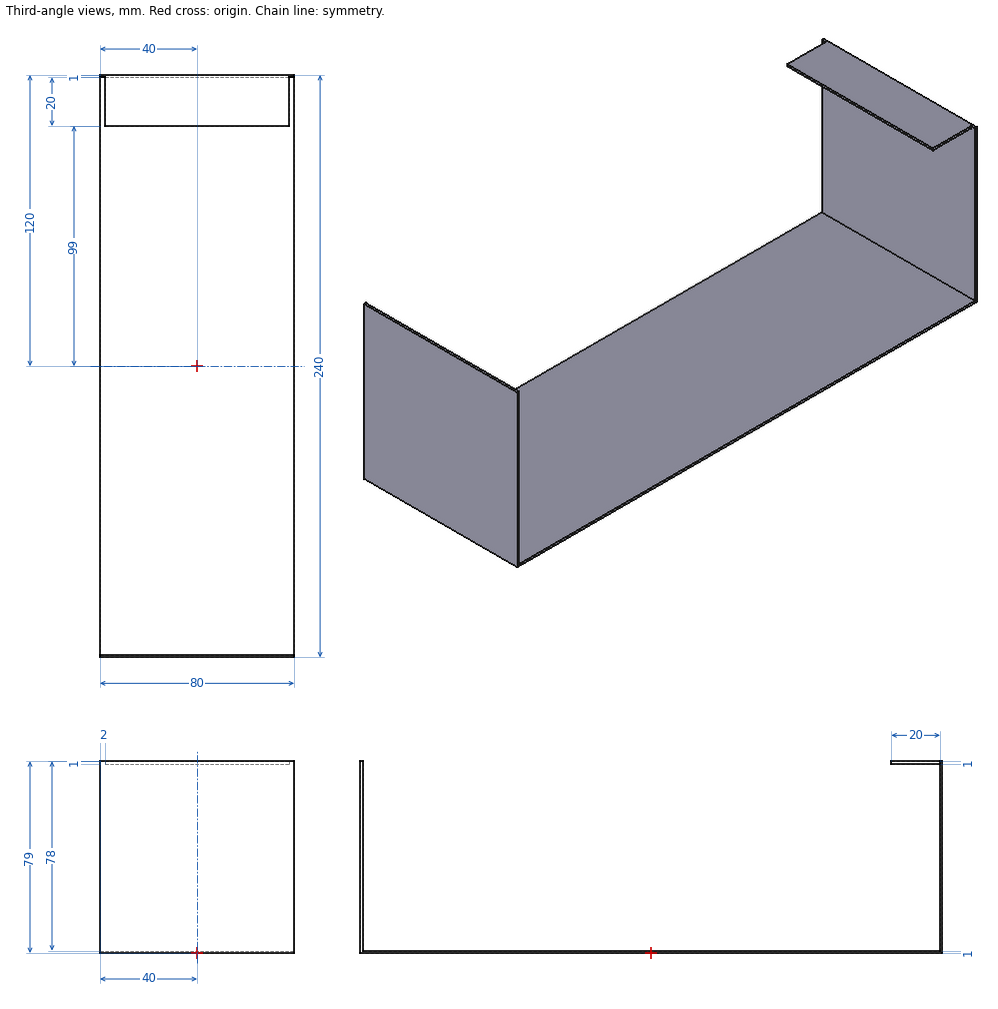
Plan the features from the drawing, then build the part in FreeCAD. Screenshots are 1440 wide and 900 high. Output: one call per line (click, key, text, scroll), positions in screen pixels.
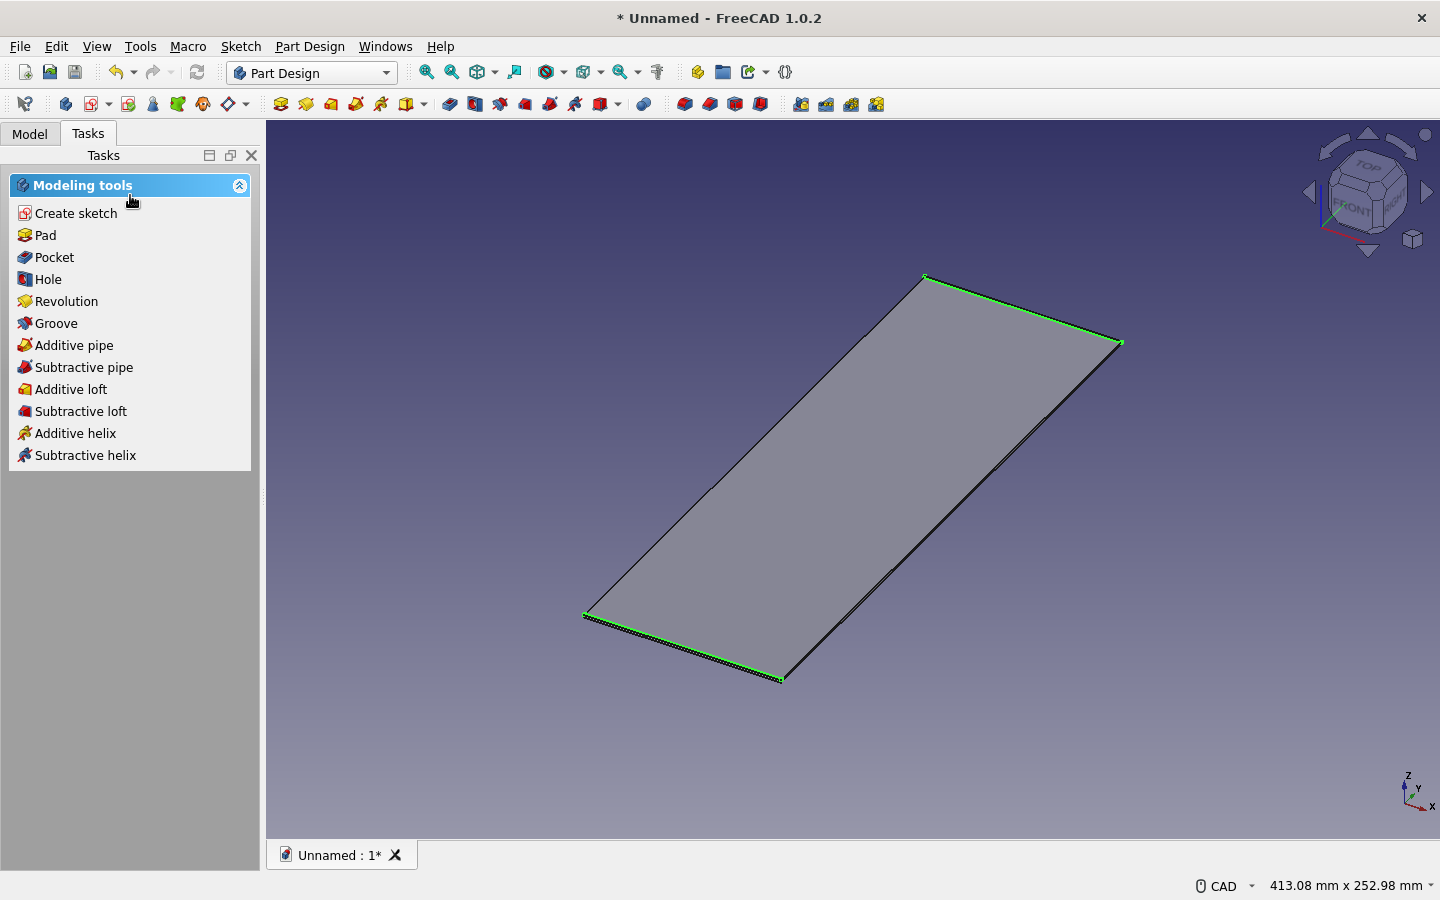
click(281, 104)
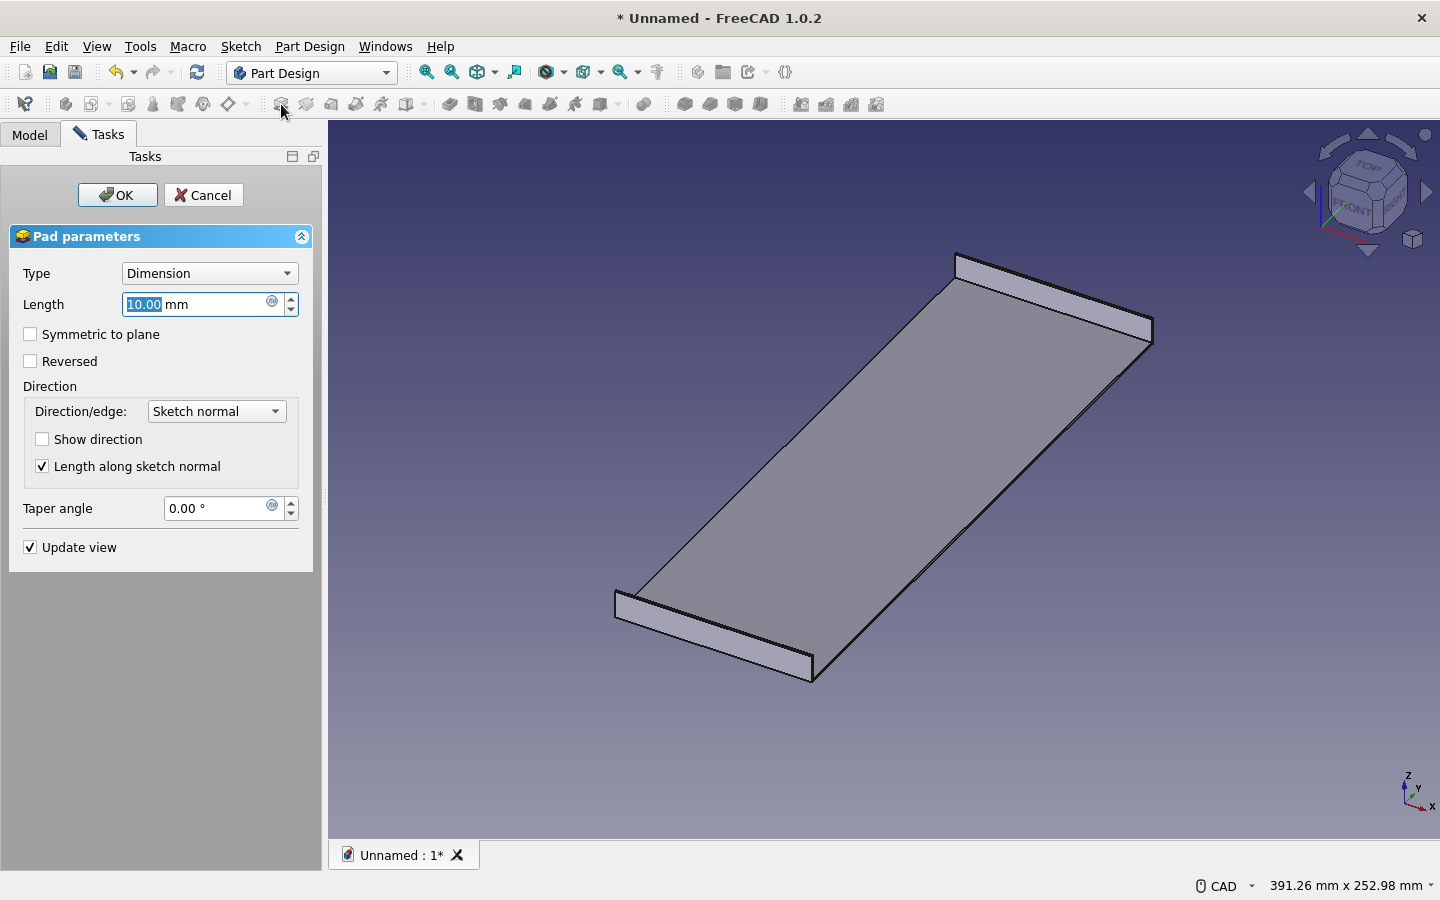
text(78)
key(Tab)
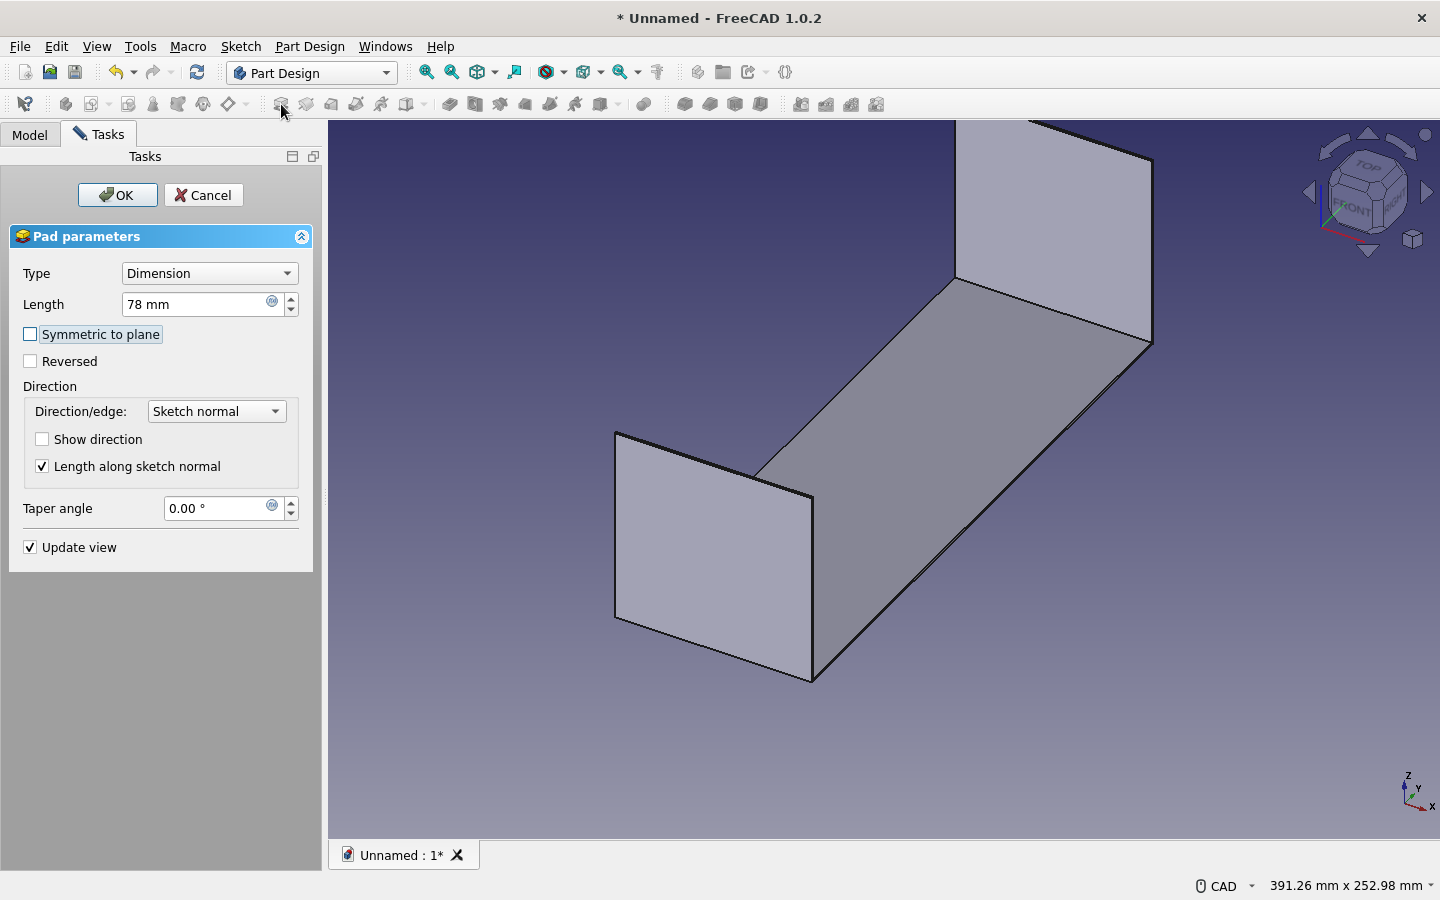
click(118, 195)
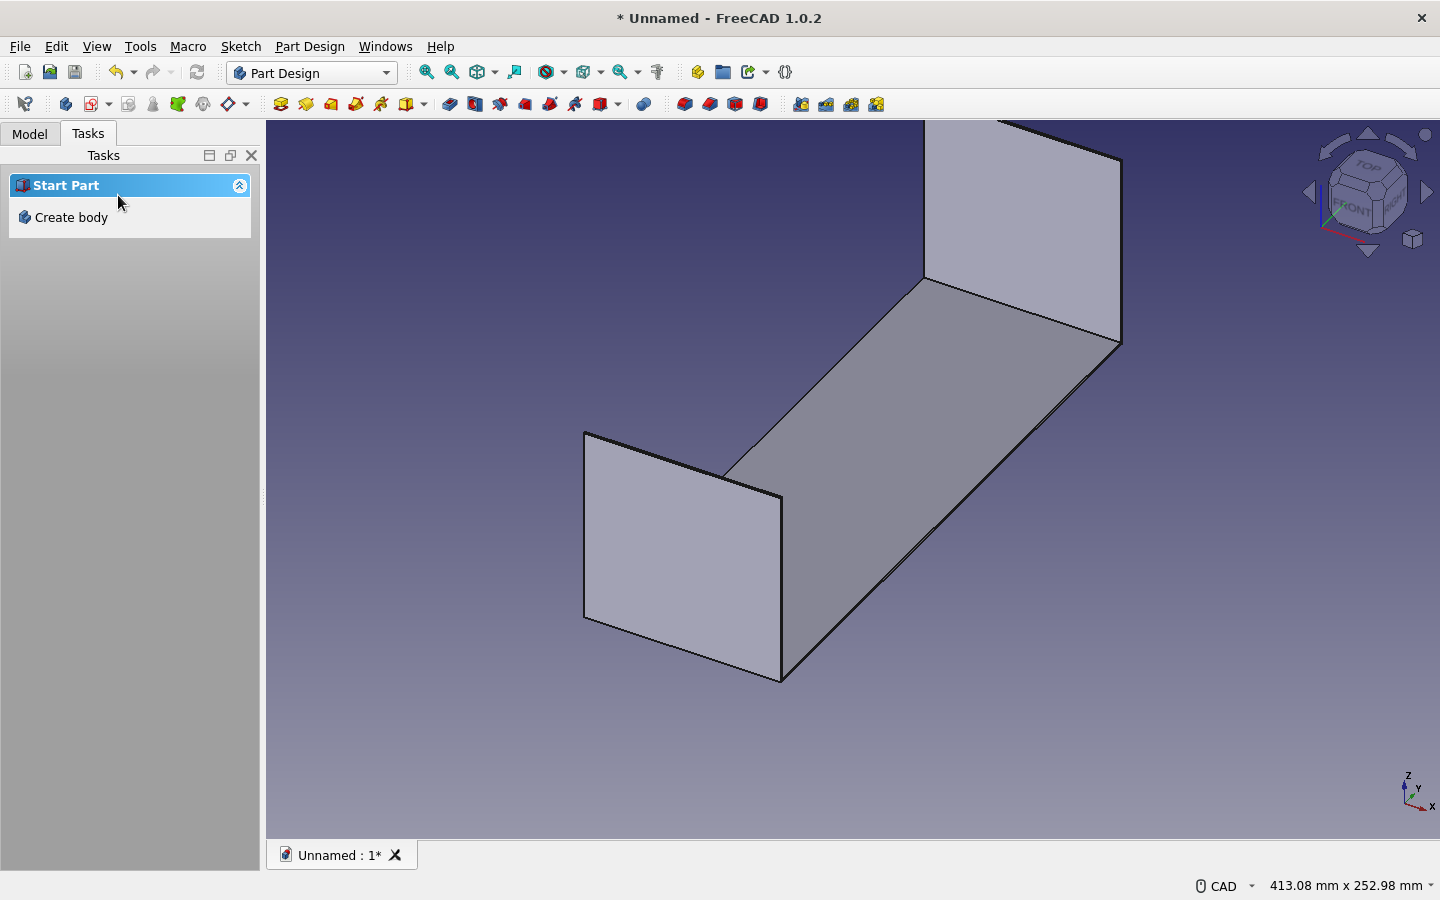
key(v)
key(f)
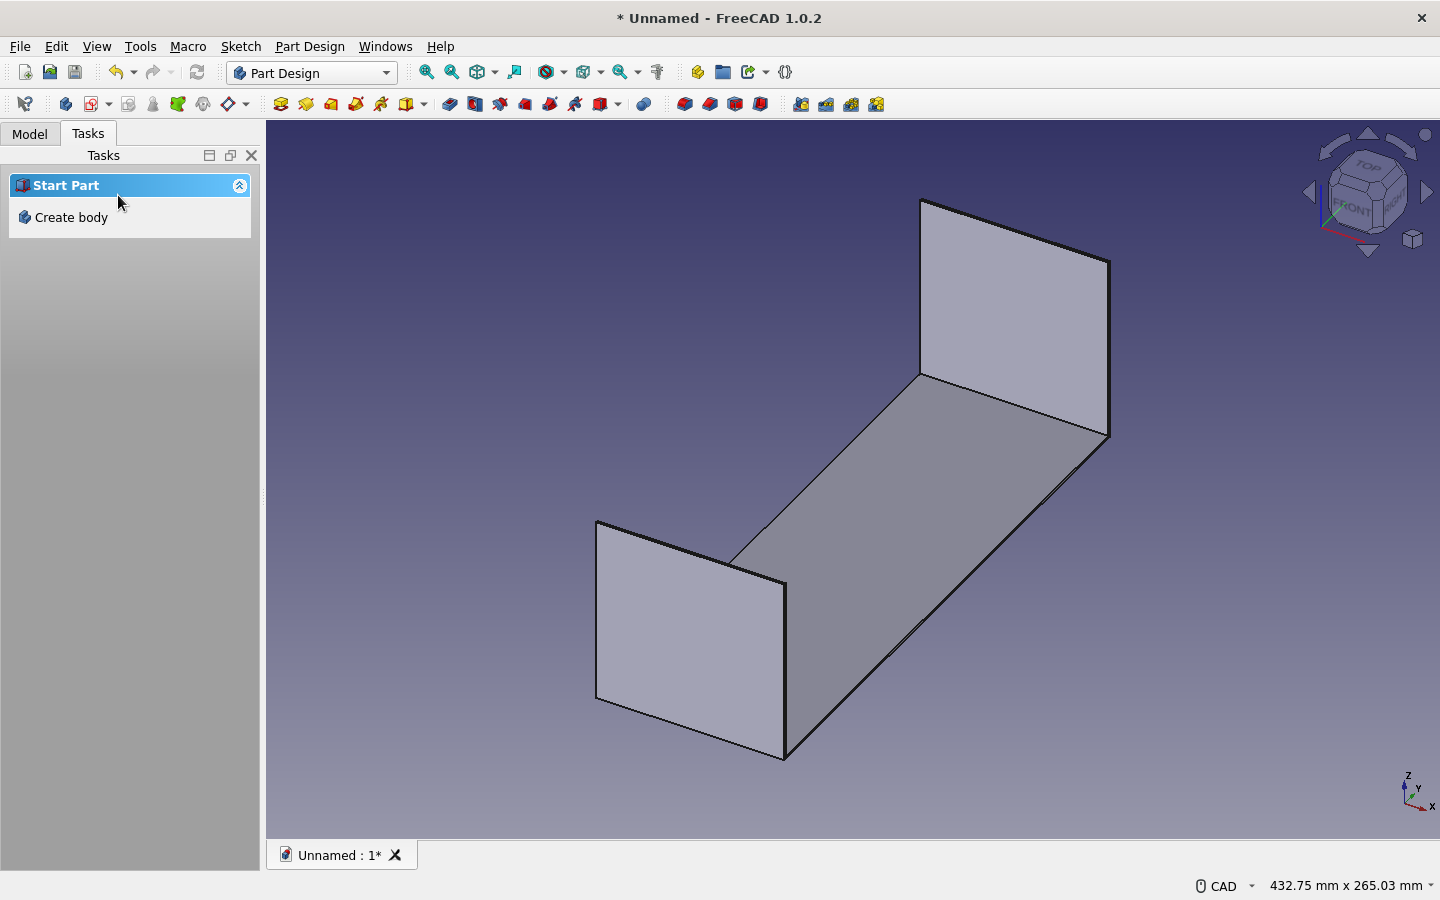
scroll(771, 578, up, 11)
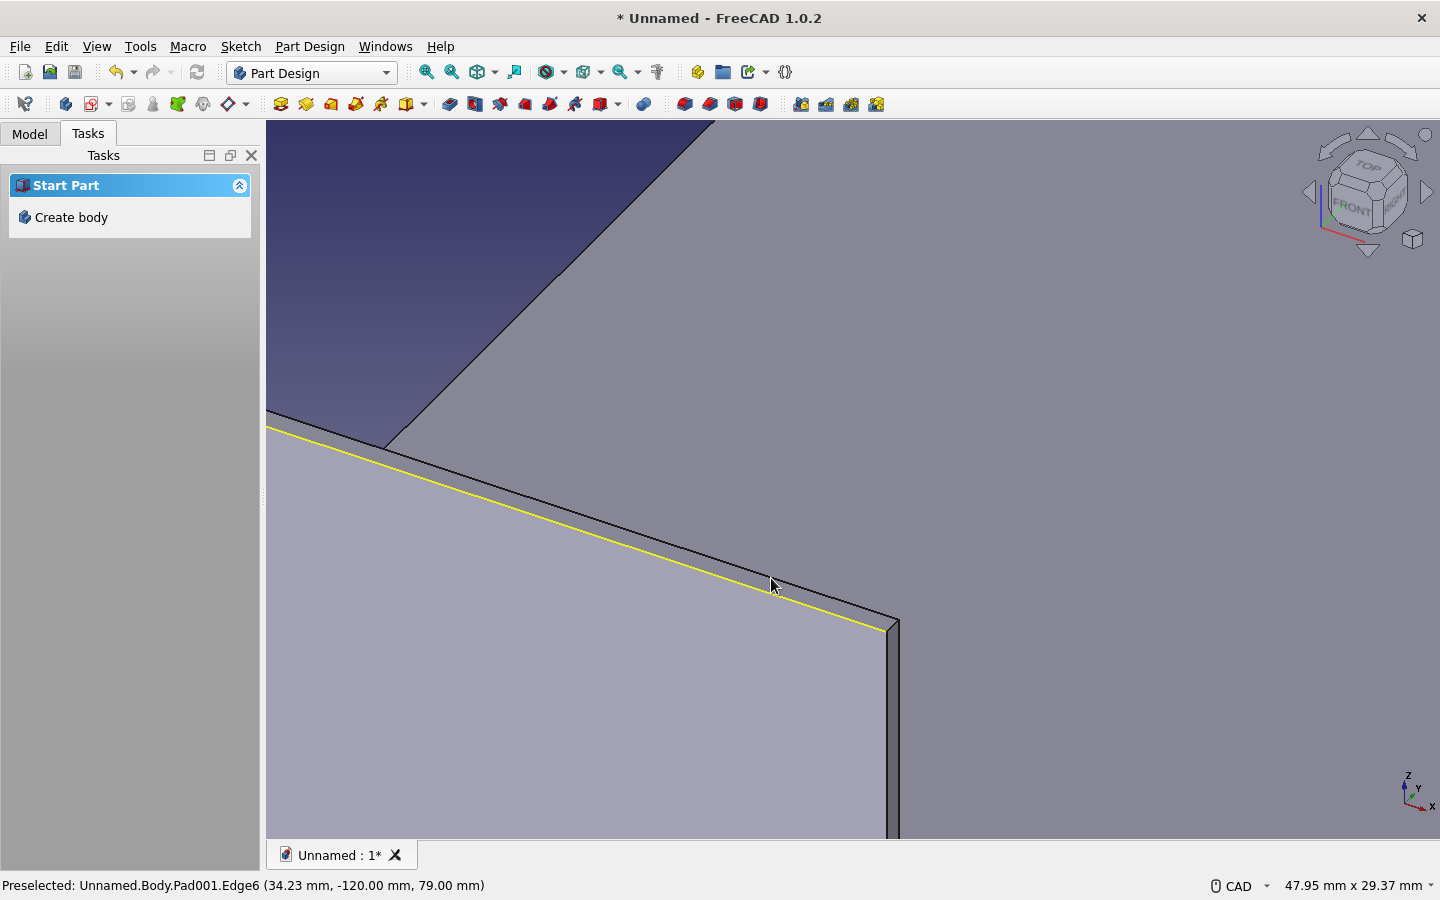
click(773, 583)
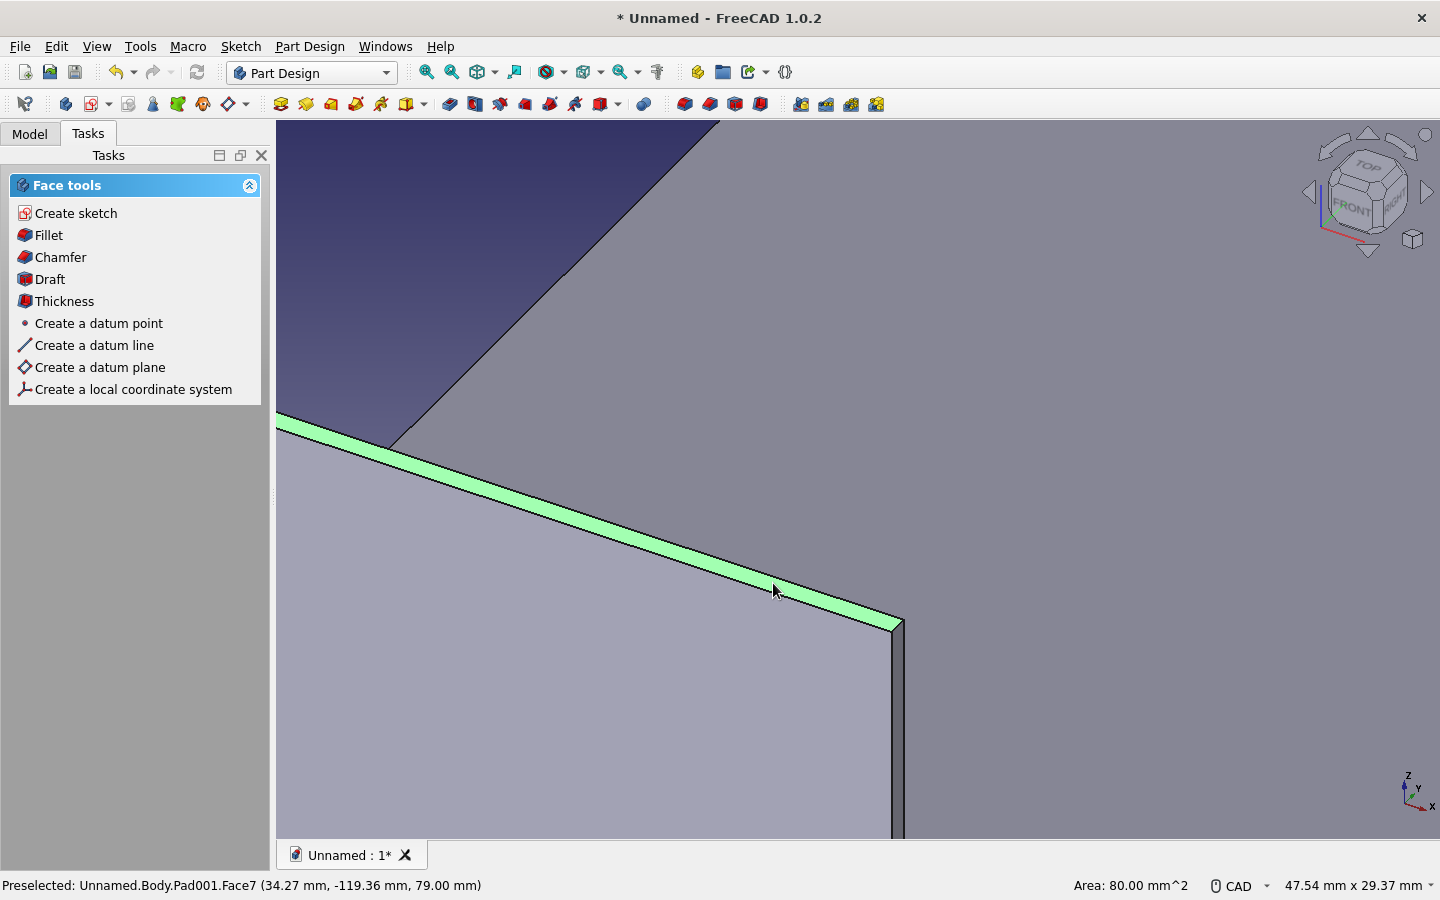
click(90, 104)